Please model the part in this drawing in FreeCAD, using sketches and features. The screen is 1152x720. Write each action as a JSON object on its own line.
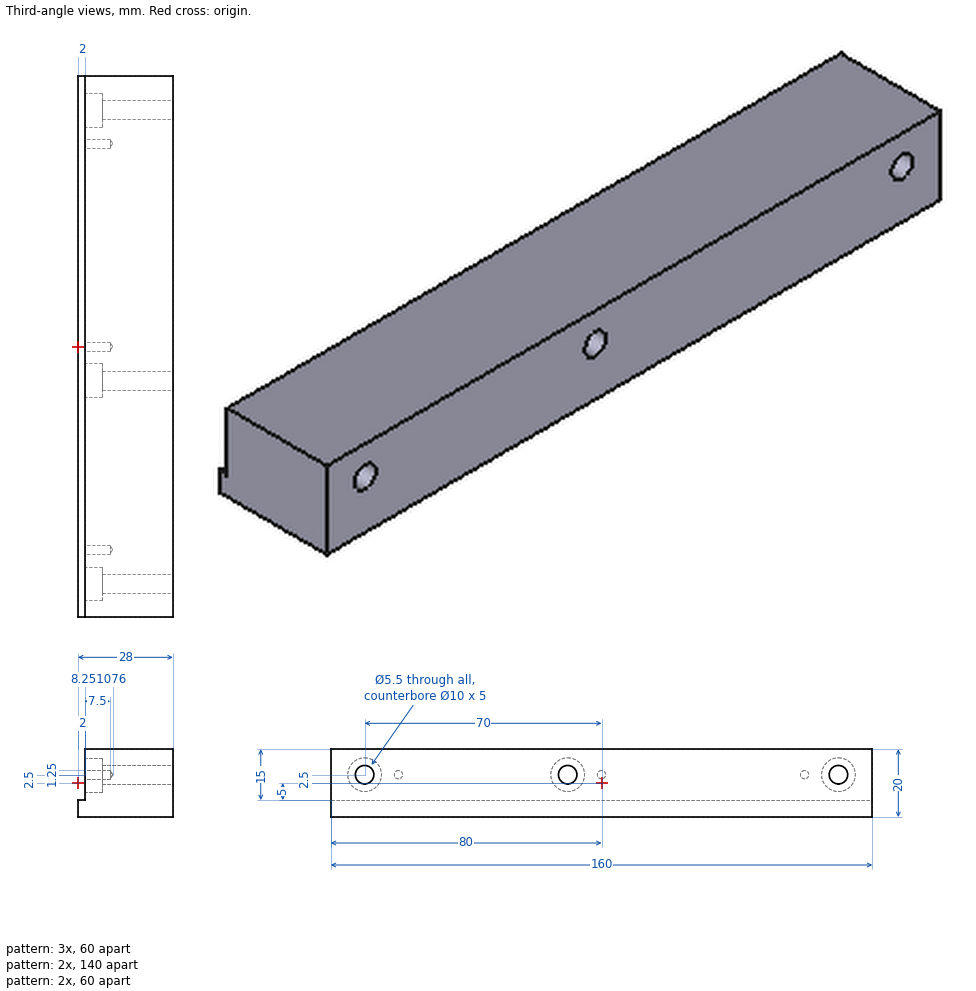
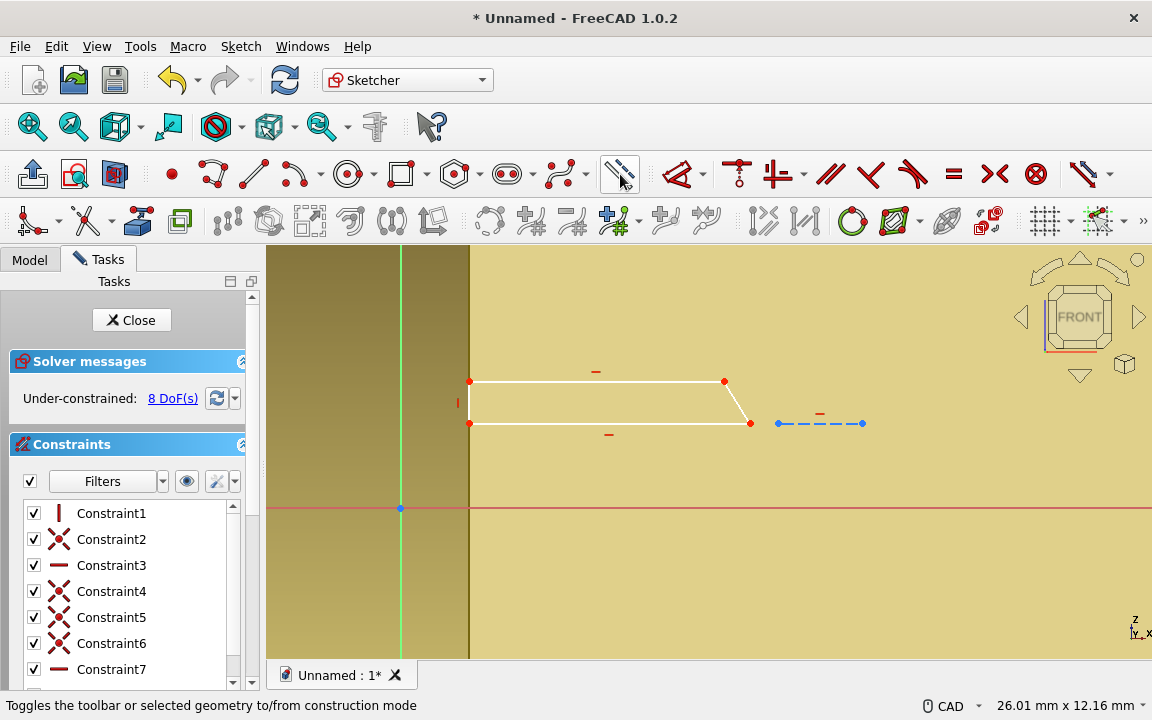
{"action": "left_click", "coordinate": [676, 174]}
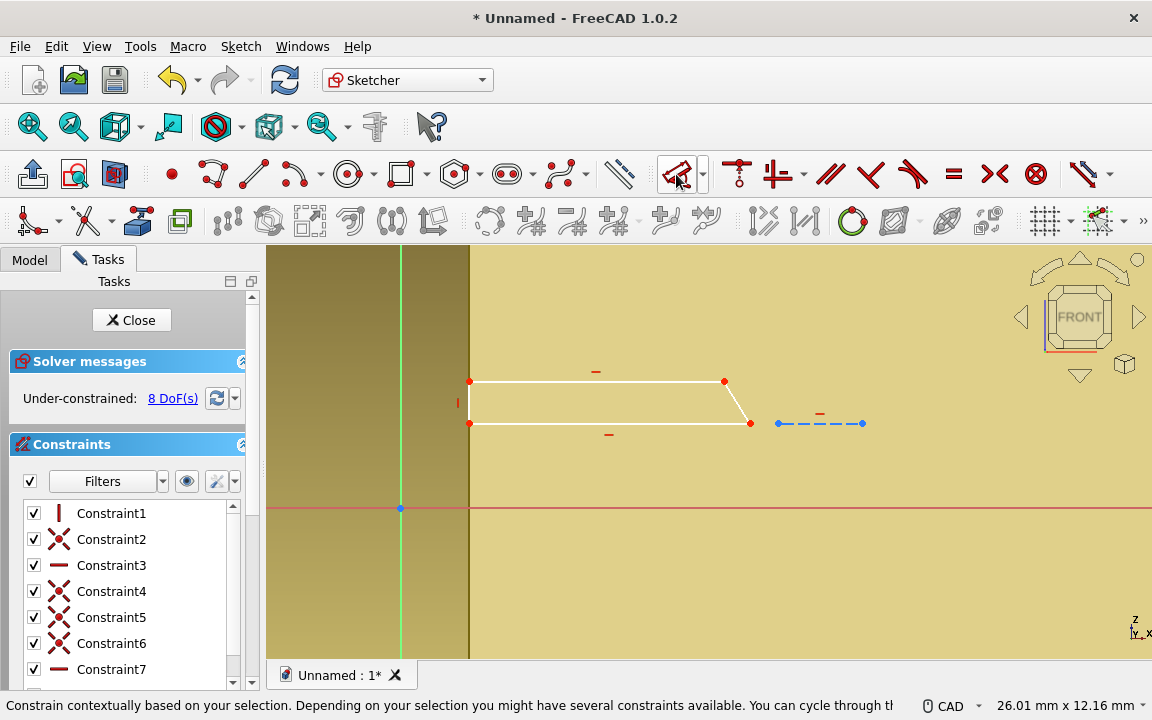
{"action": "left_click", "coordinate": [469, 424]}
{"action": "left_click", "coordinate": [435, 542]}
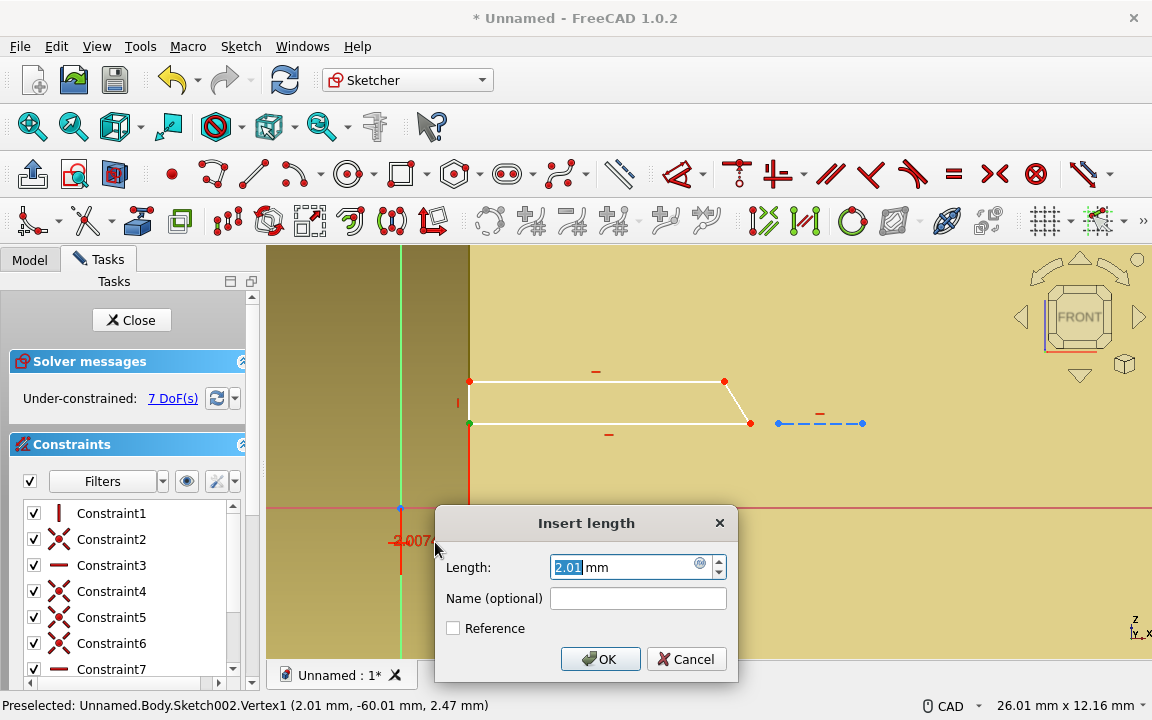
{"action": "type", "text": "2"}
{"action": "key", "text": "Return"}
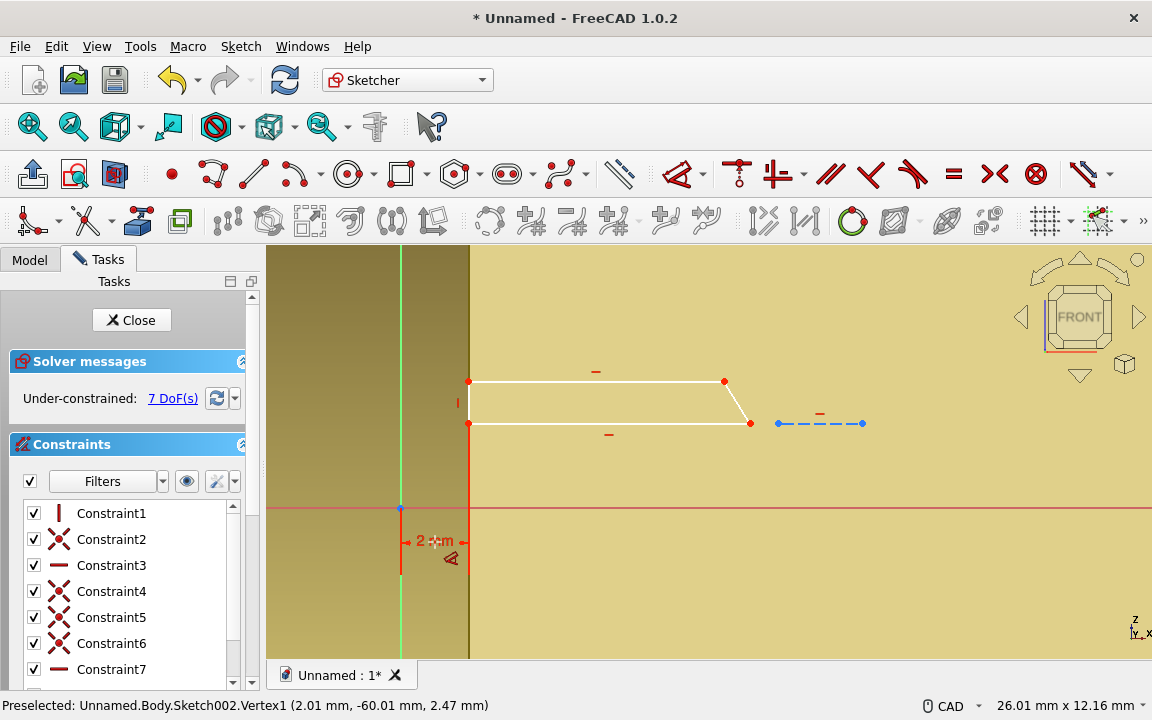
{"action": "left_click", "coordinate": [545, 382]}
{"action": "left_click", "coordinate": [596, 348]}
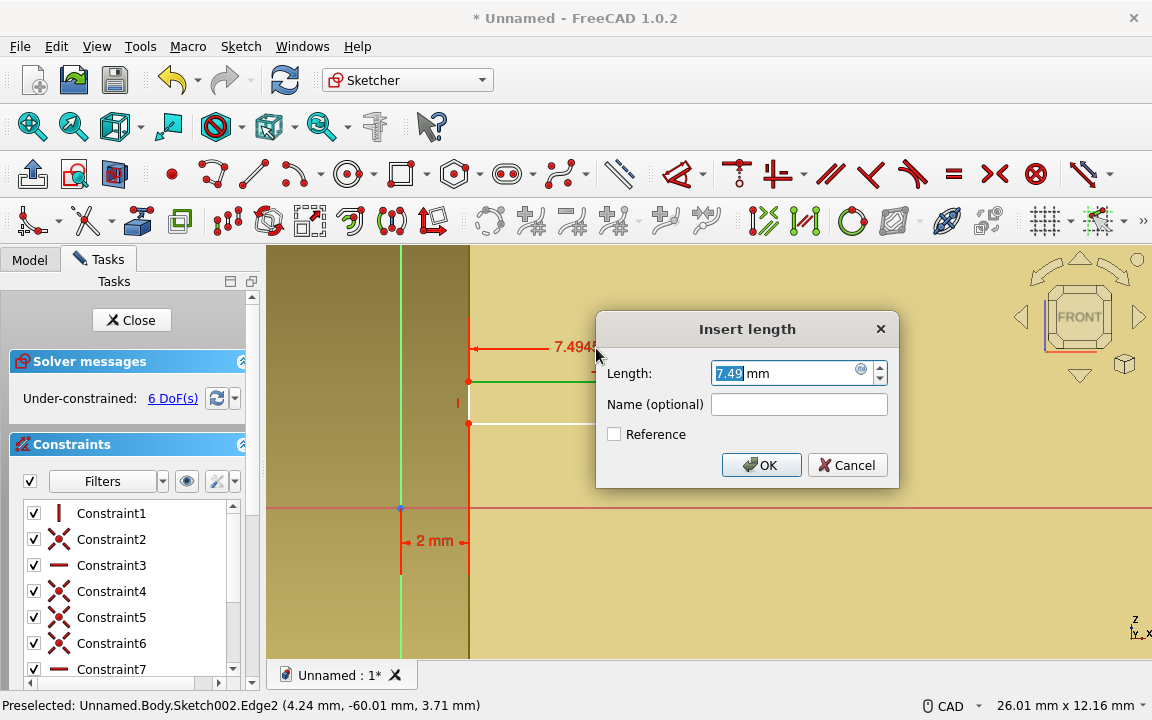
{"action": "type", "text": "7.5"}
{"action": "key", "text": "Return"}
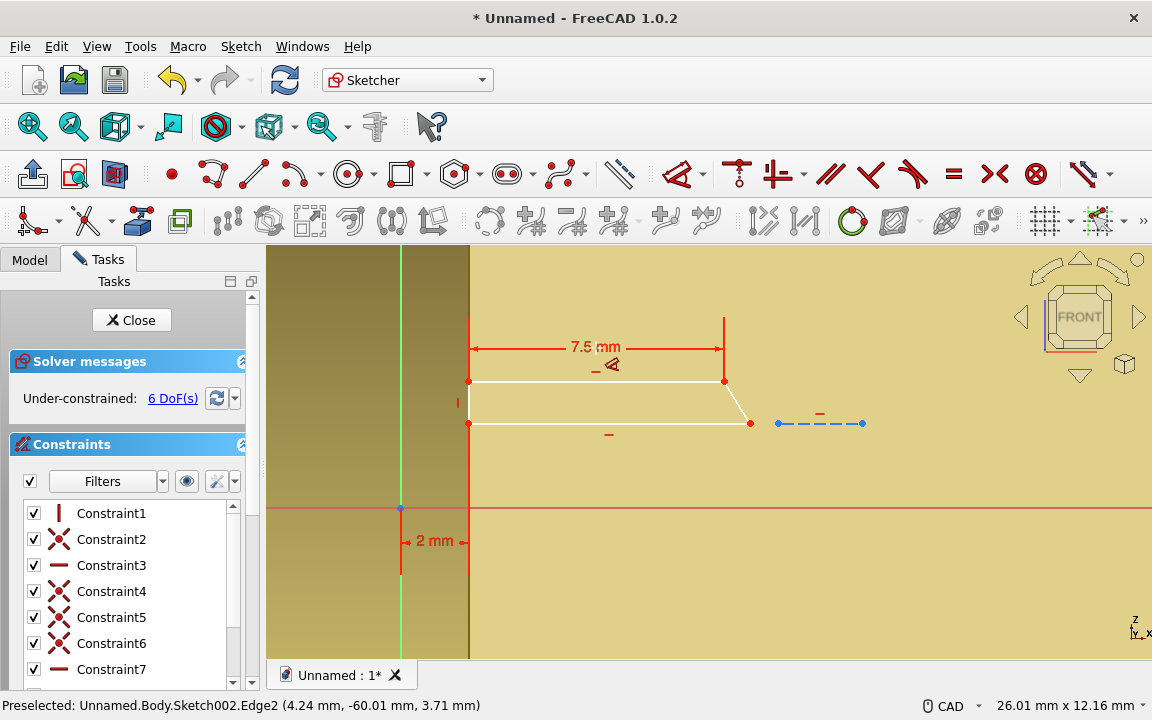
{"action": "left_click", "coordinate": [469, 411]}
{"action": "left_click", "coordinate": [435, 403]}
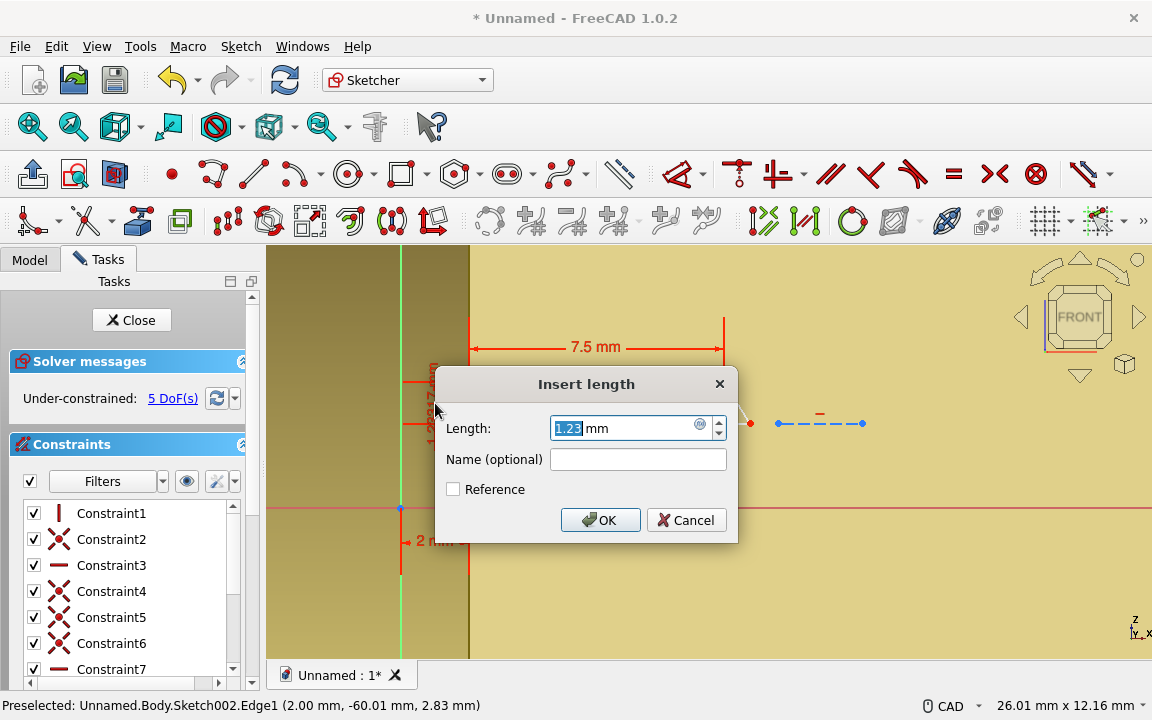
{"action": "type", "text": "1.25"}
{"action": "key", "text": "Return"}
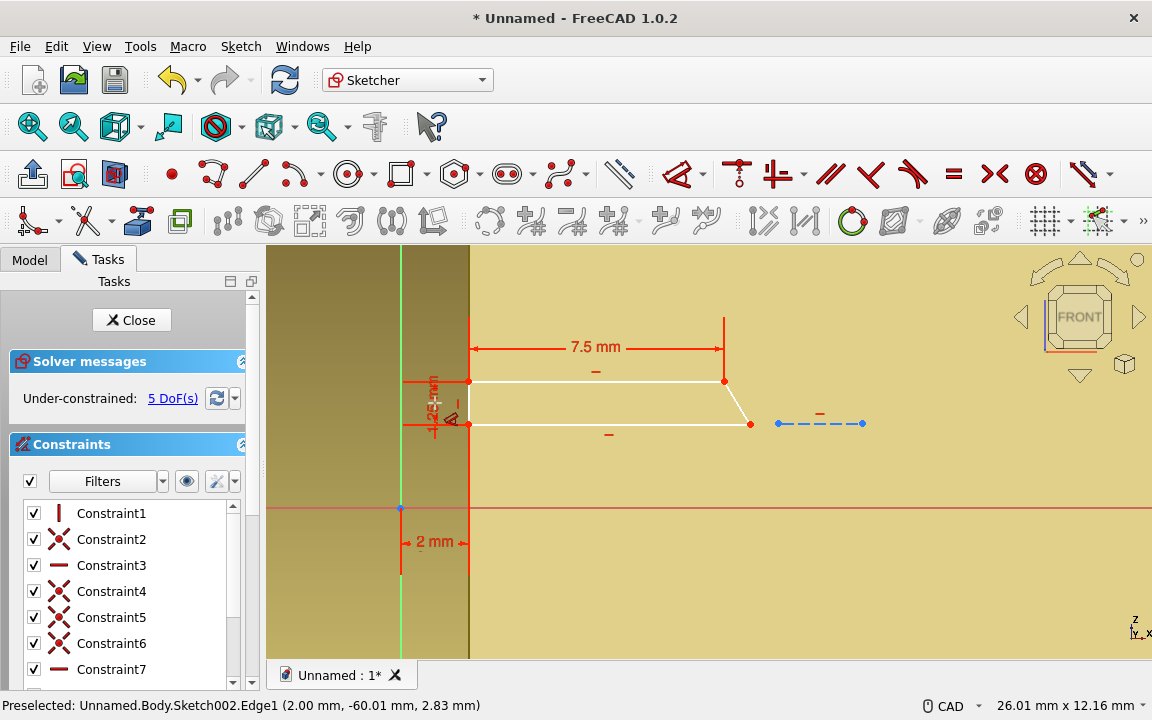
{"action": "left_click", "coordinate": [469, 425]}
{"action": "left_click", "coordinate": [367, 466]}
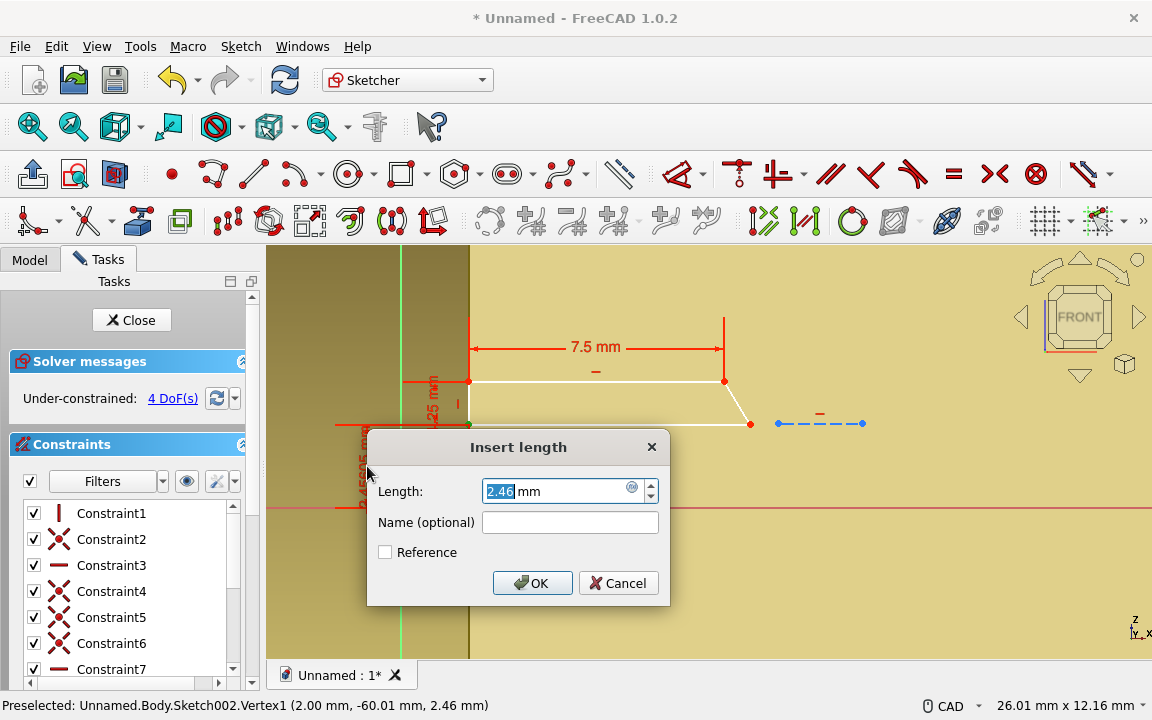
{"action": "type", "text": "2.5"}
{"action": "key", "text": "Return"}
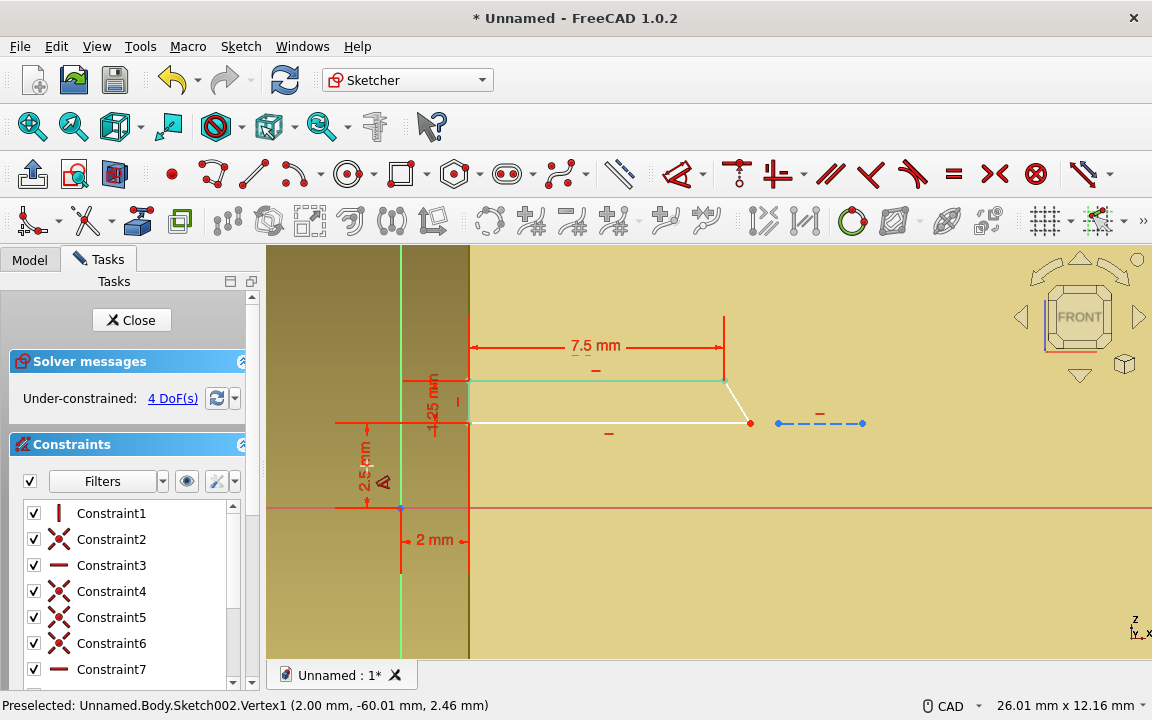
{"action": "left_click", "coordinate": [778, 424]}
{"action": "left_click", "coordinate": [367, 437]}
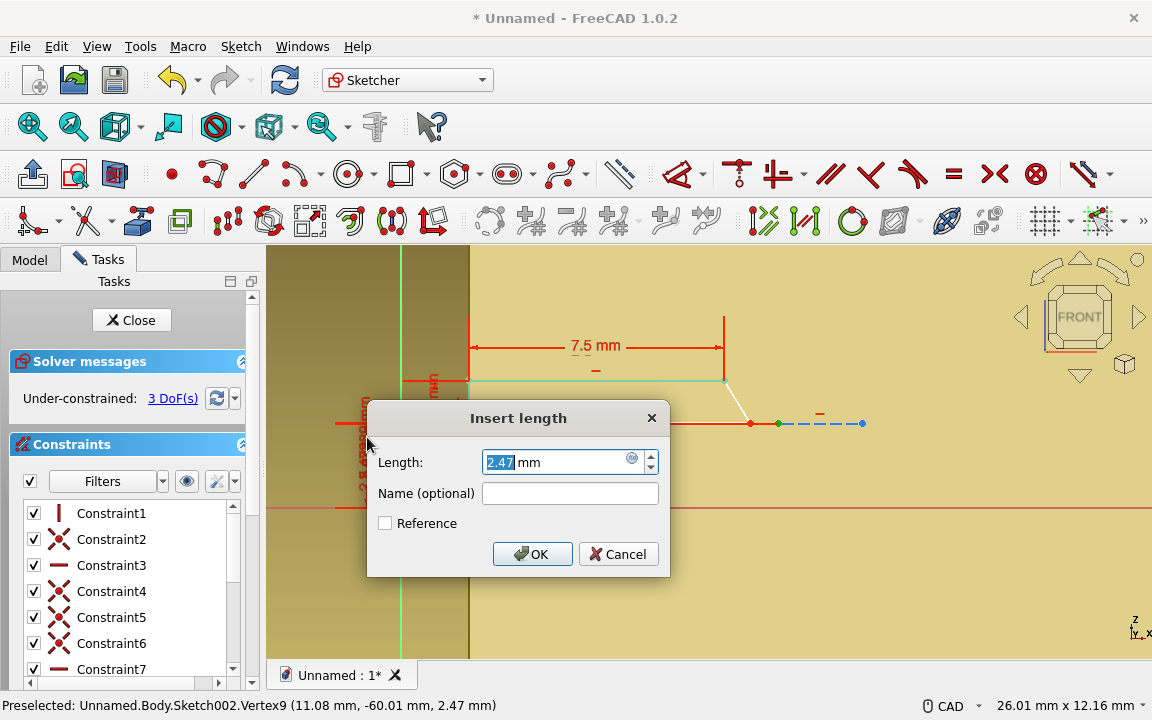
{"action": "type", "text": "2.5"}
{"action": "key", "text": "Return"}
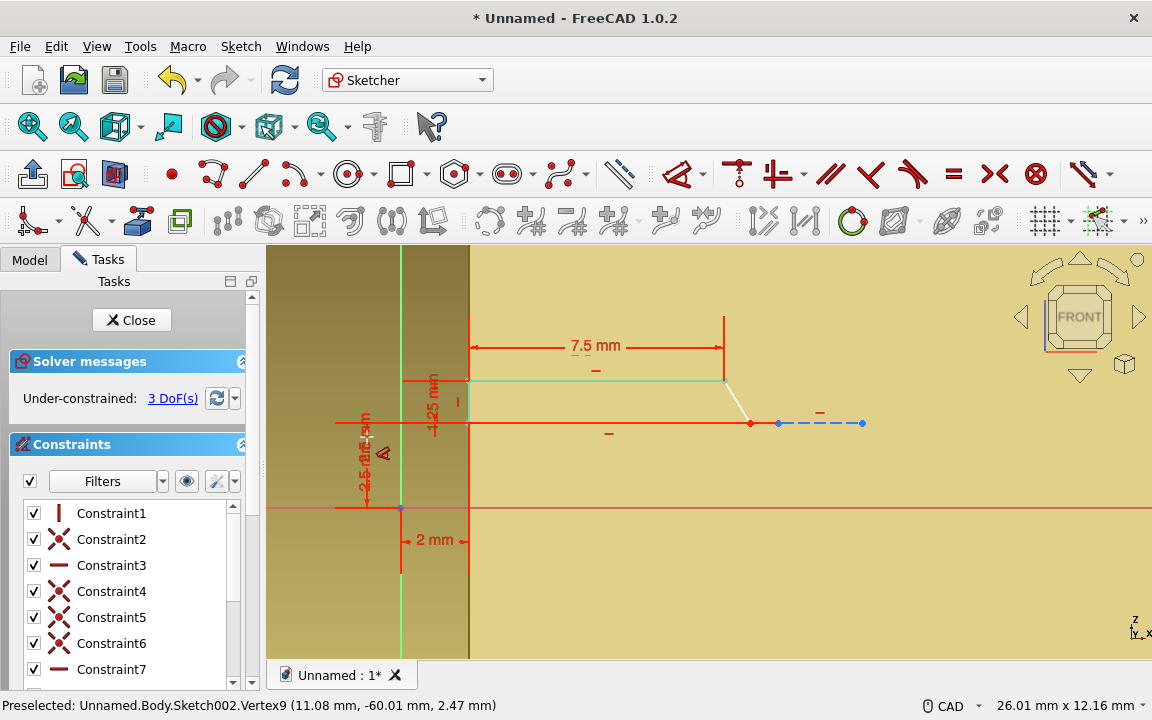
{"action": "left_click", "coordinate": [666, 423]}
{"action": "left_click", "coordinate": [609, 457]}